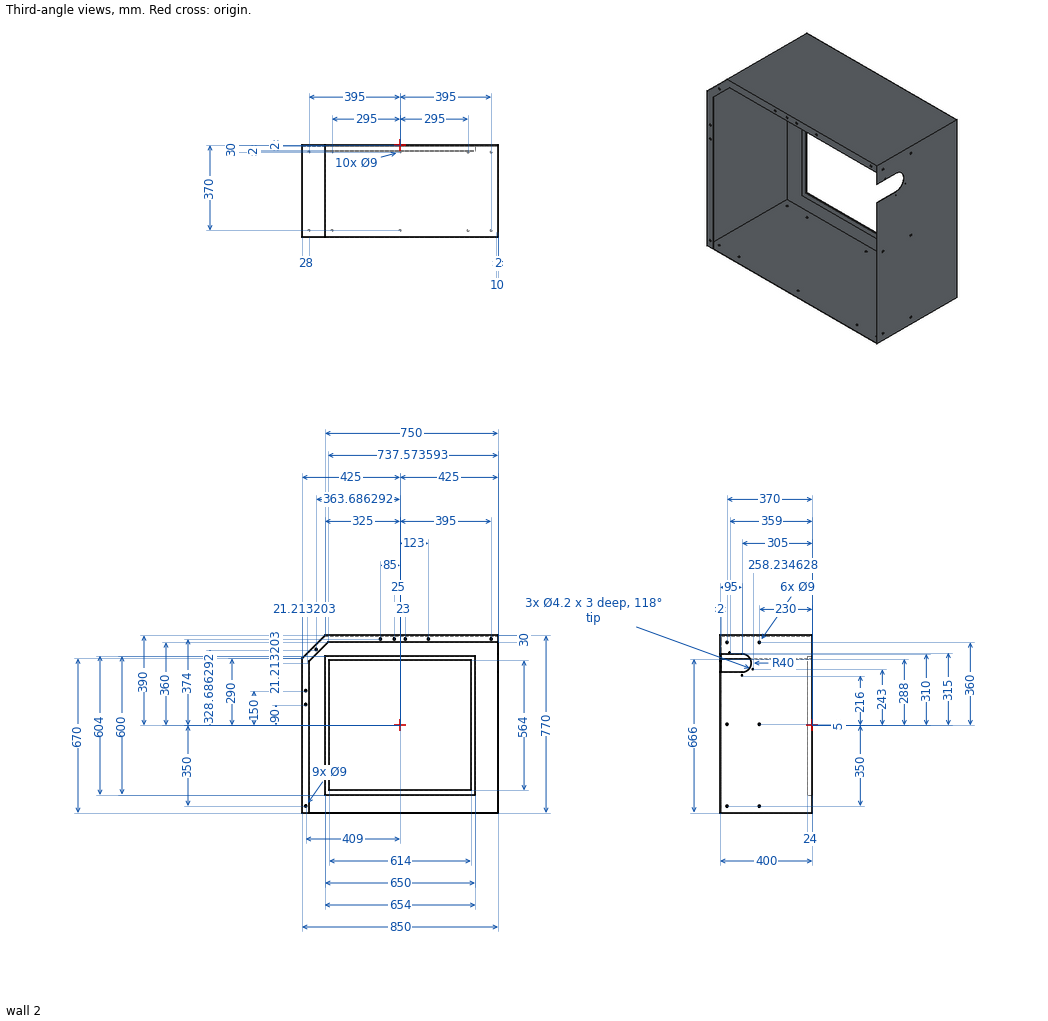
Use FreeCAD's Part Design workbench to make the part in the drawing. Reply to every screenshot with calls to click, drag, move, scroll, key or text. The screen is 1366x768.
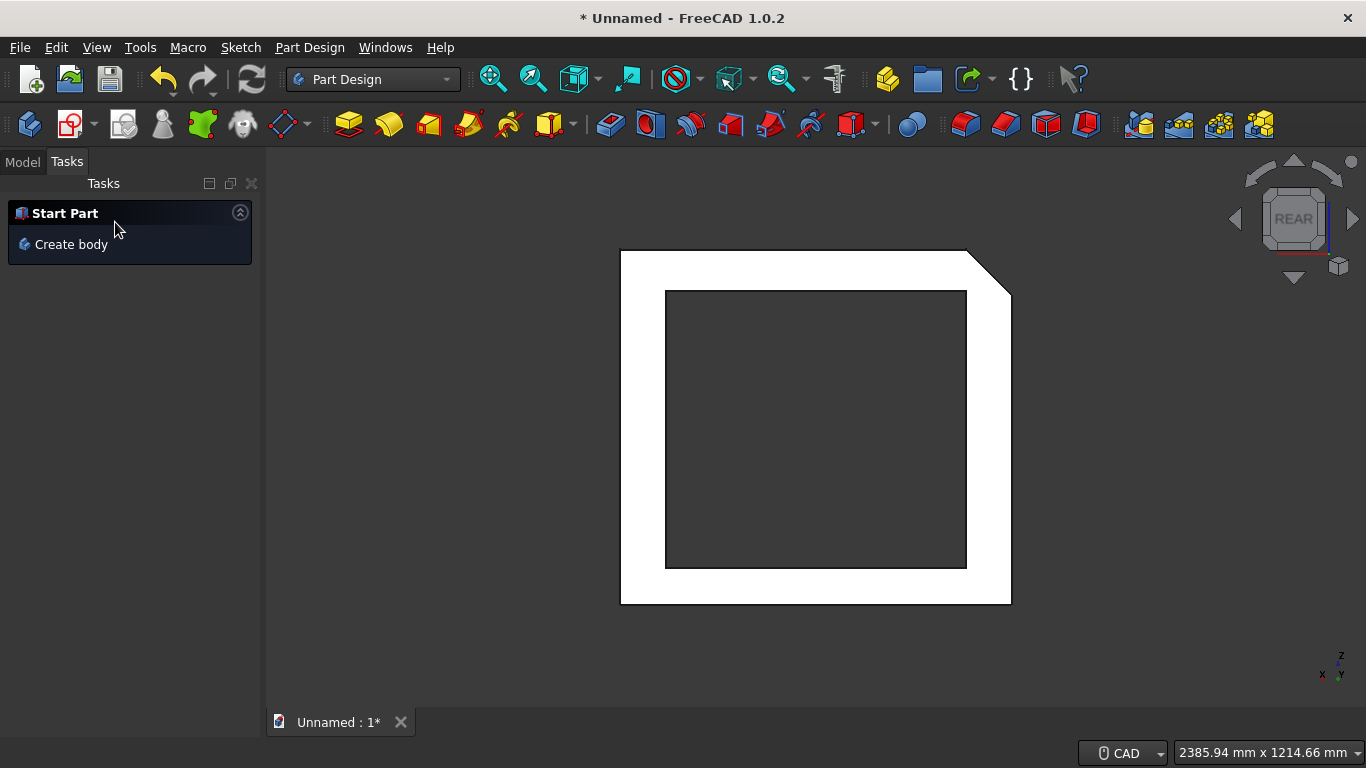
key(0)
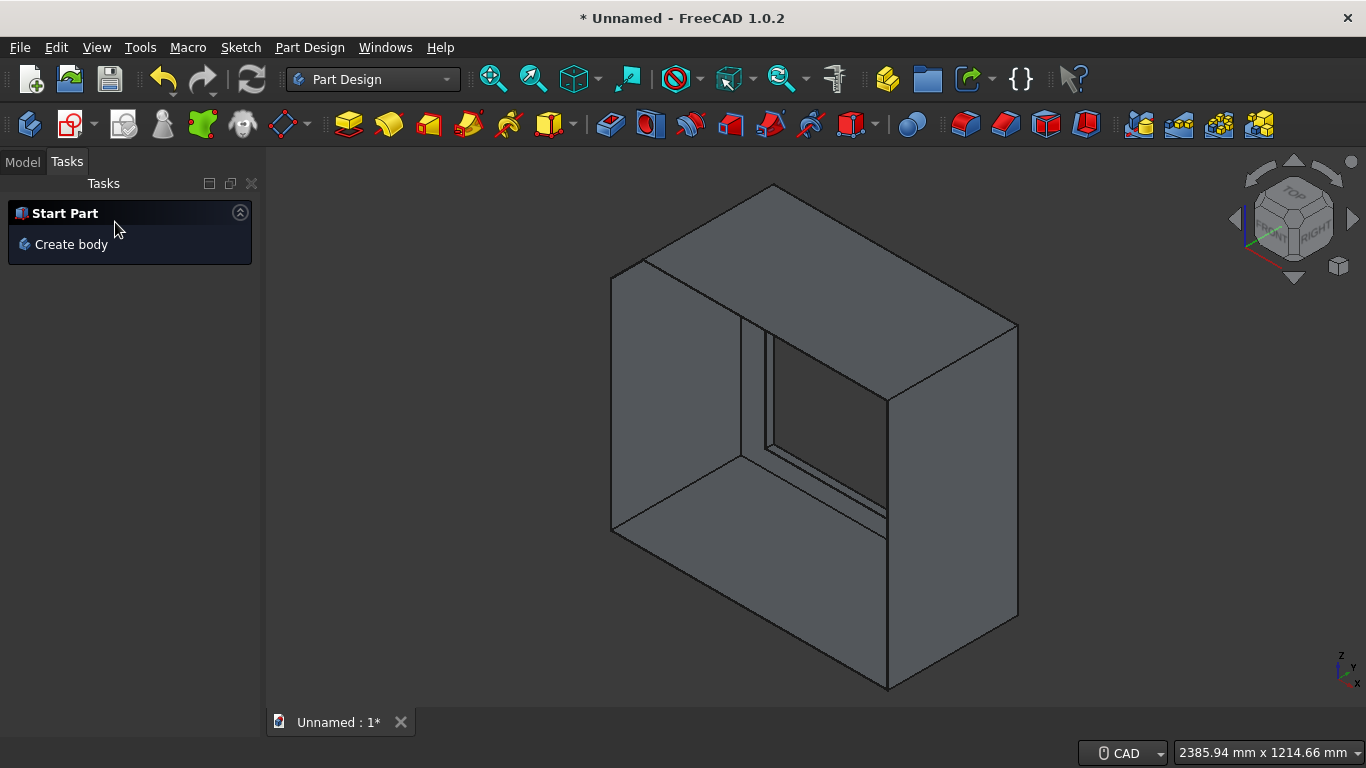
scroll(978, 495, up, 15)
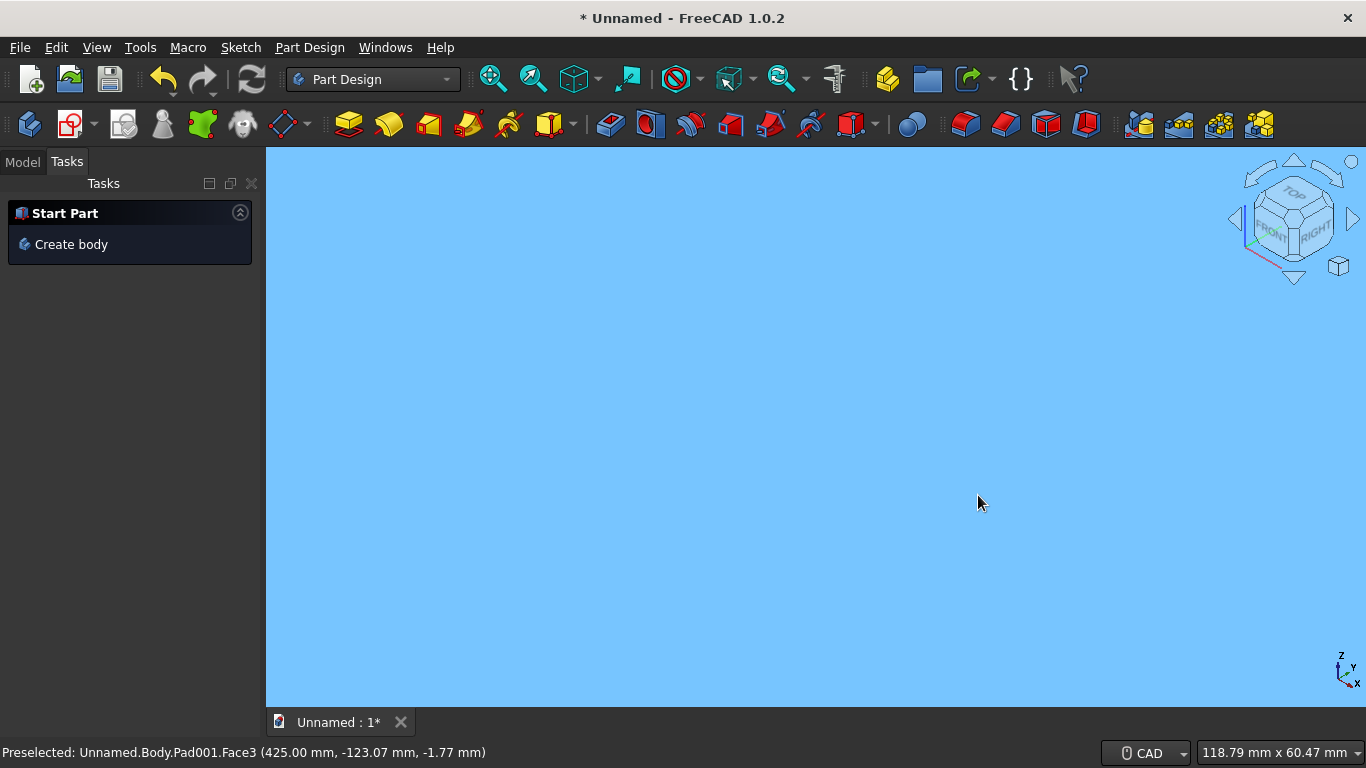
scroll(968, 497, up, 4)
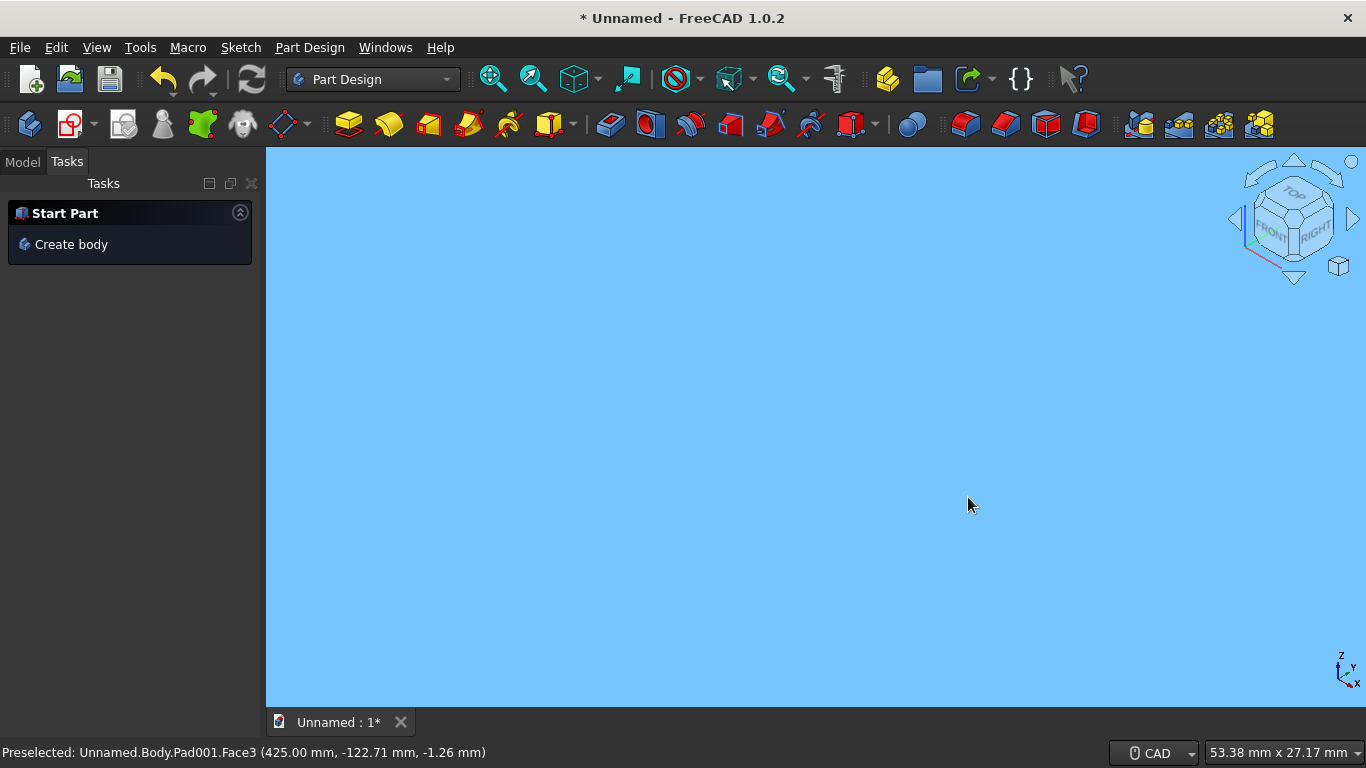
click(494, 80)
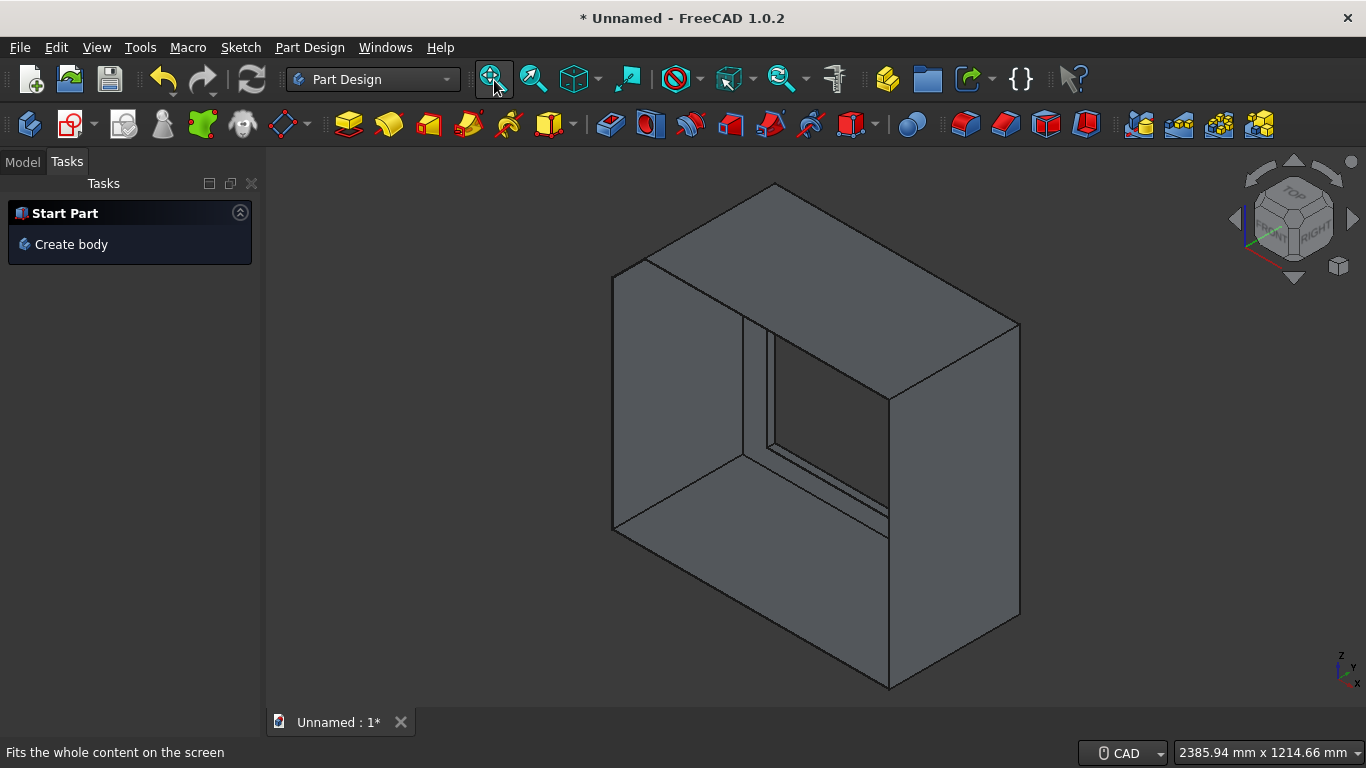
key(1)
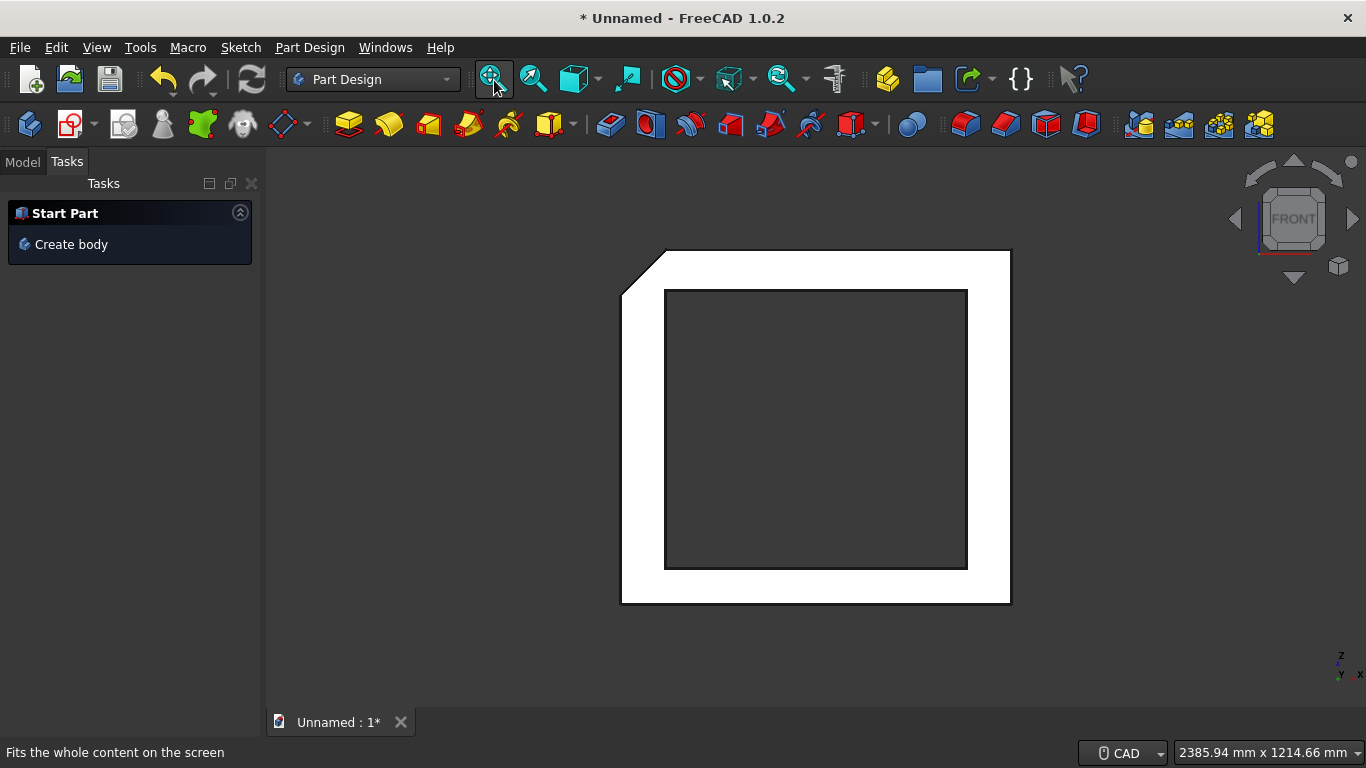
scroll(966, 474, up, 15)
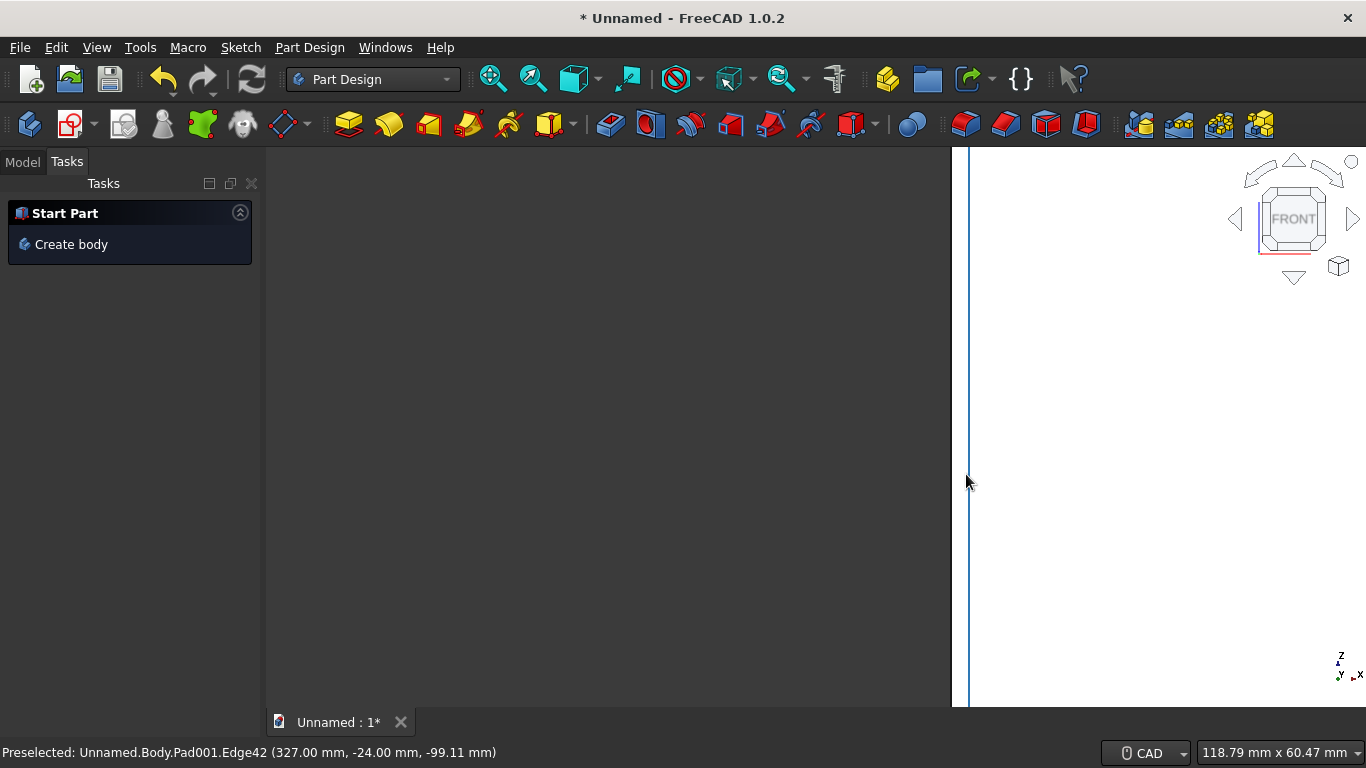
scroll(963, 490, up, 4)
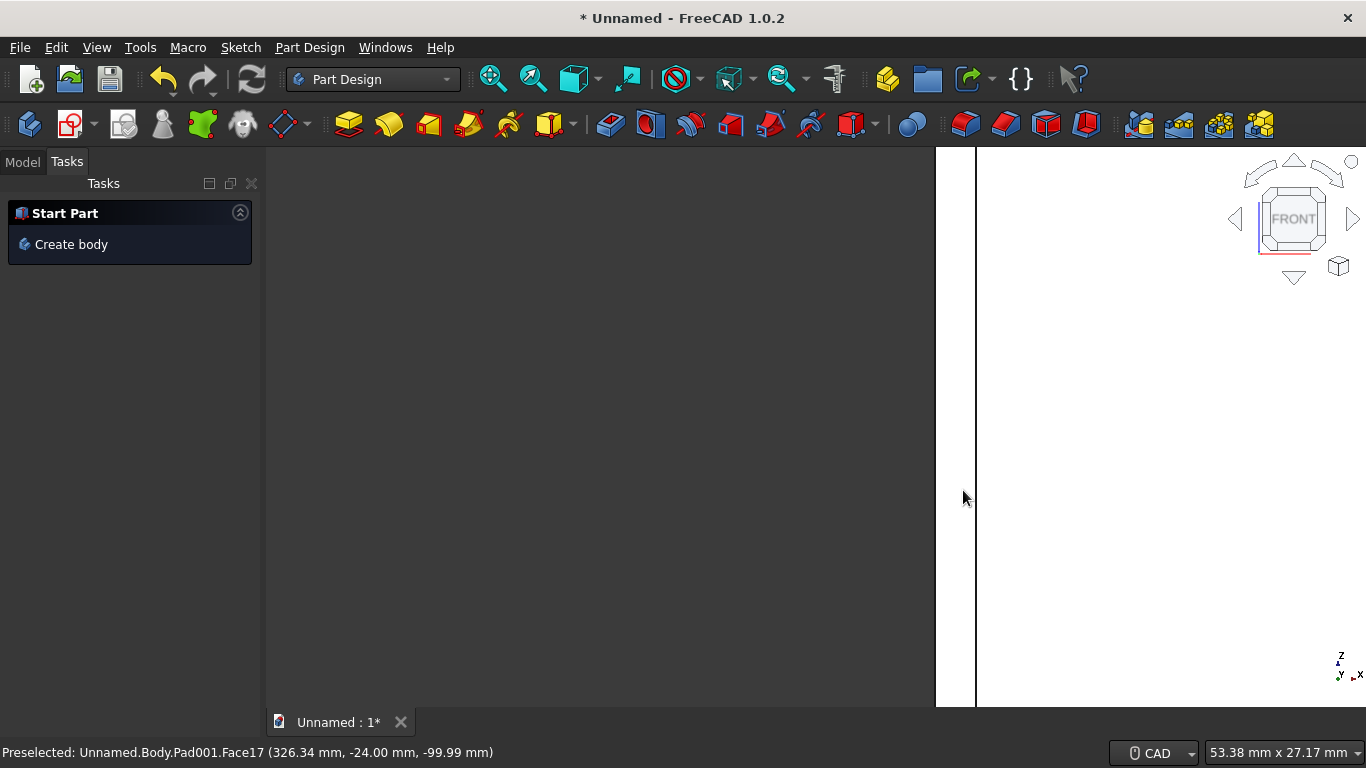
click(962, 491)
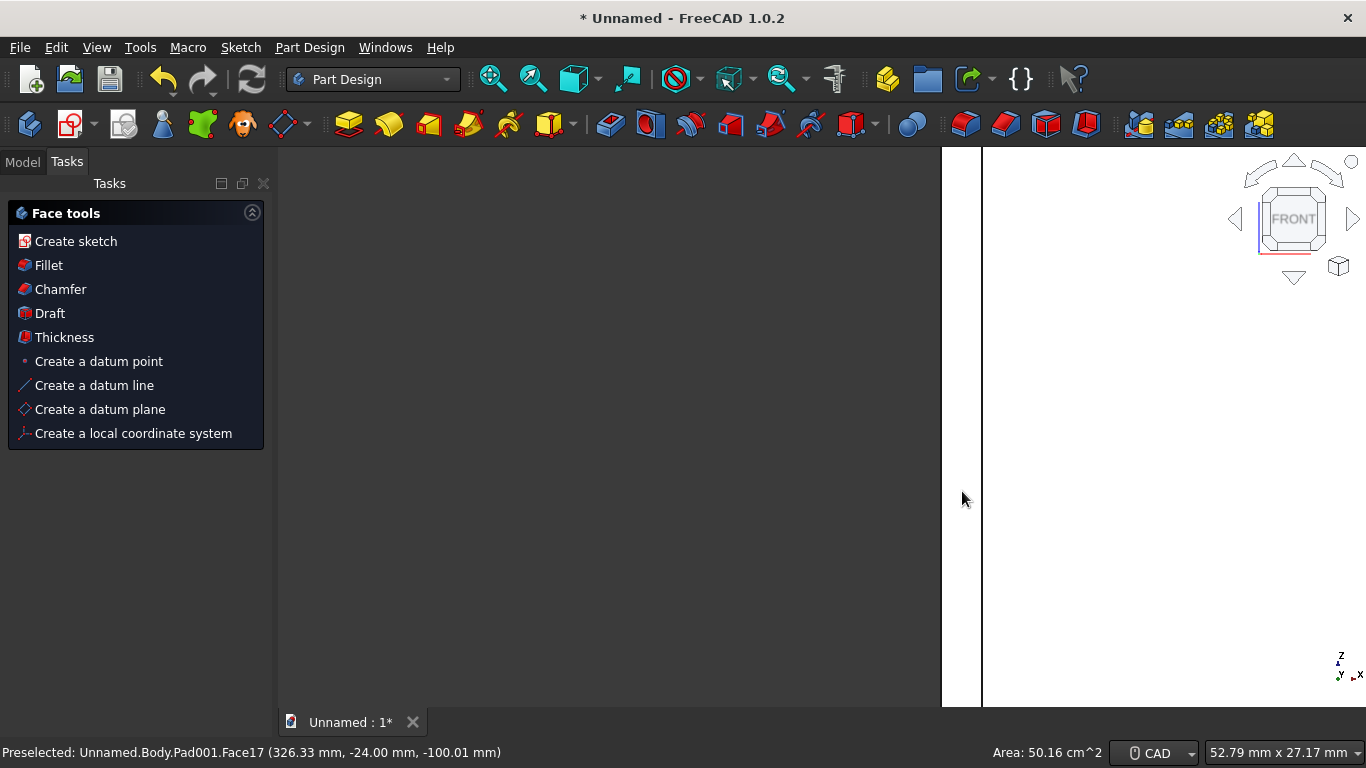
click(70, 124)